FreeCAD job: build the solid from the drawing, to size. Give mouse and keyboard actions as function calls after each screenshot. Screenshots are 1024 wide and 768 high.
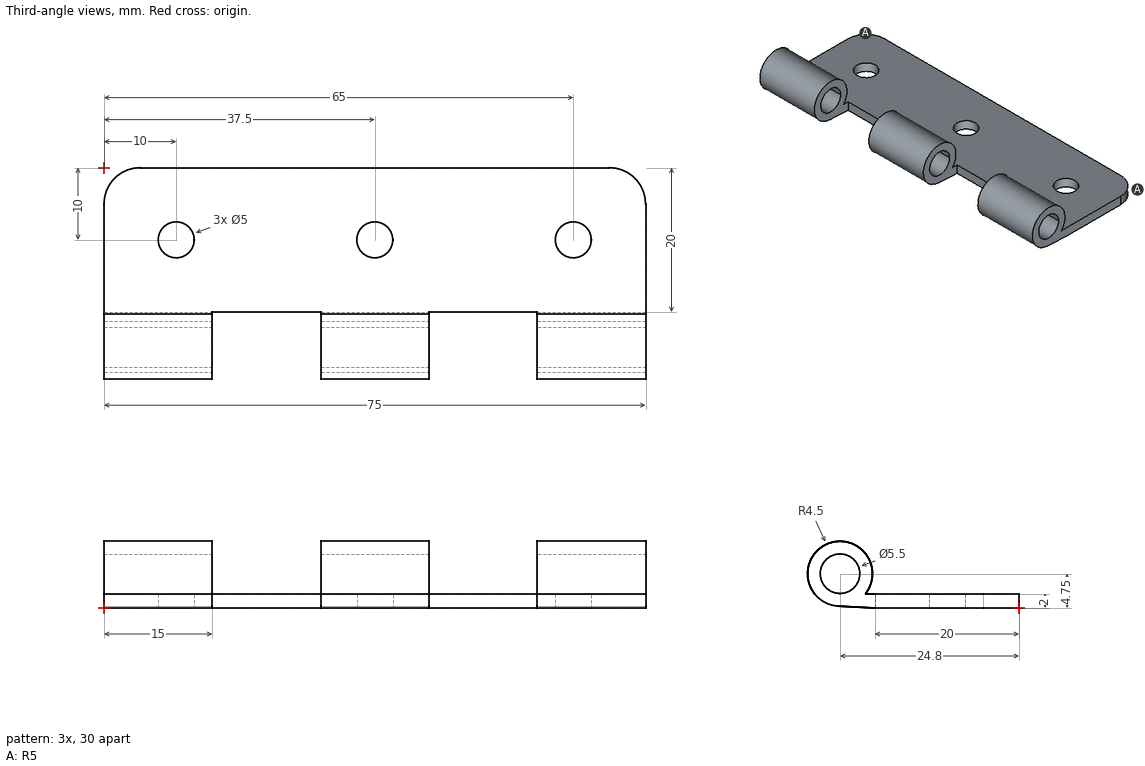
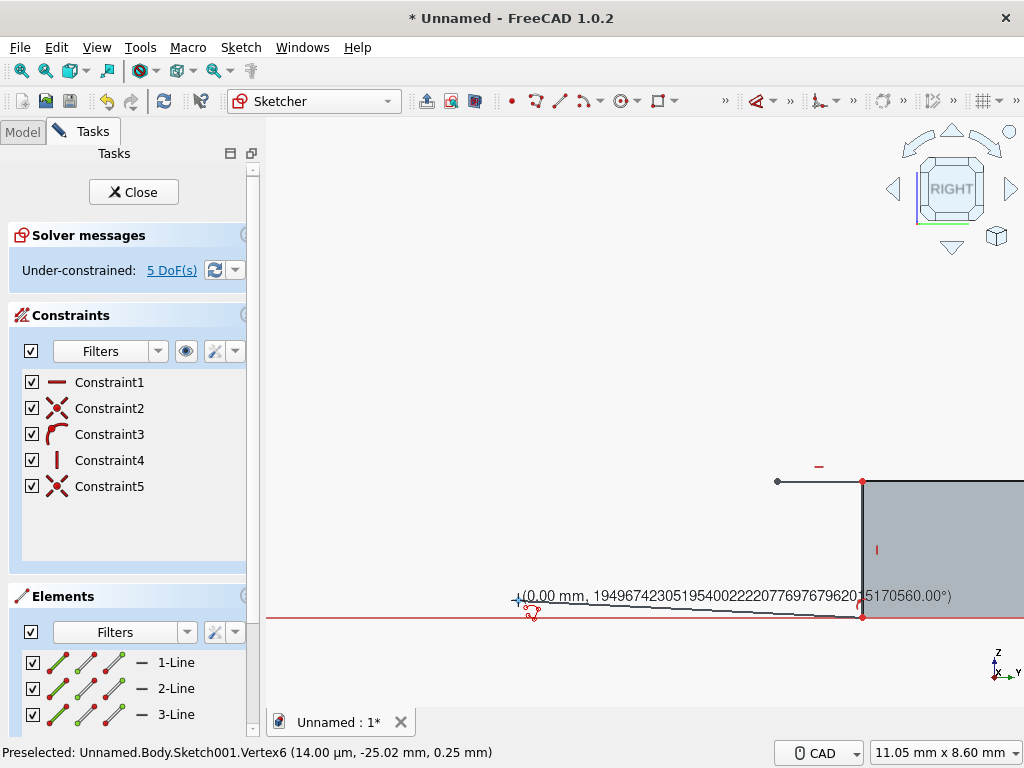
key(g)
key(3)
key(a)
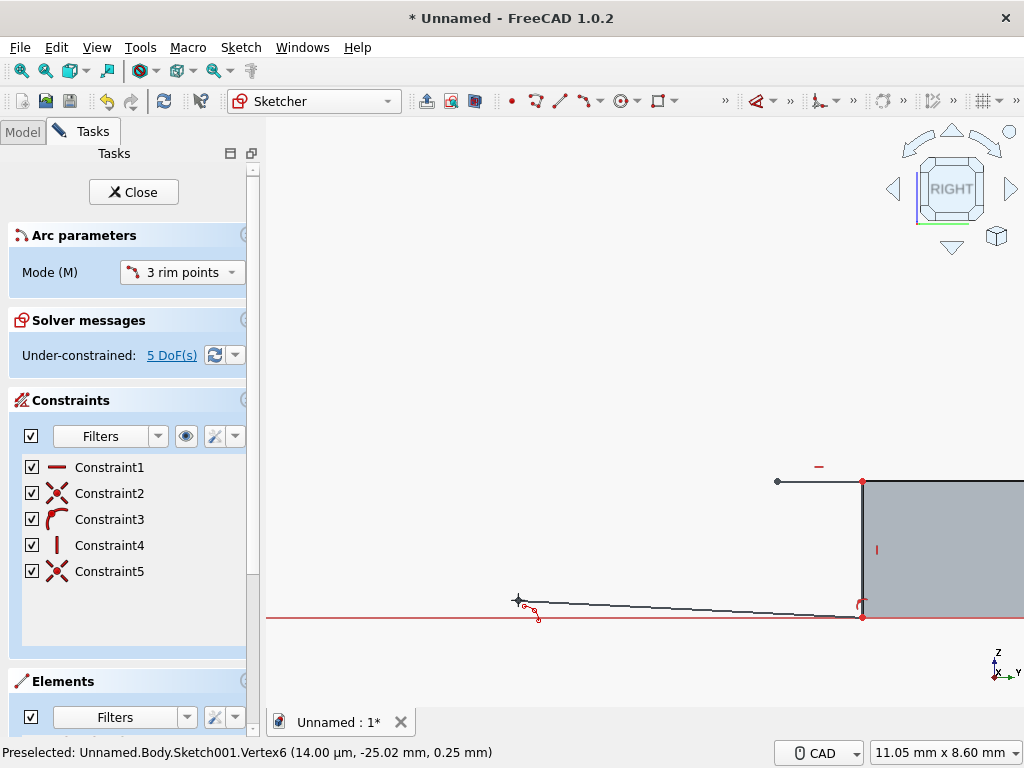
click(518, 601)
click(777, 482)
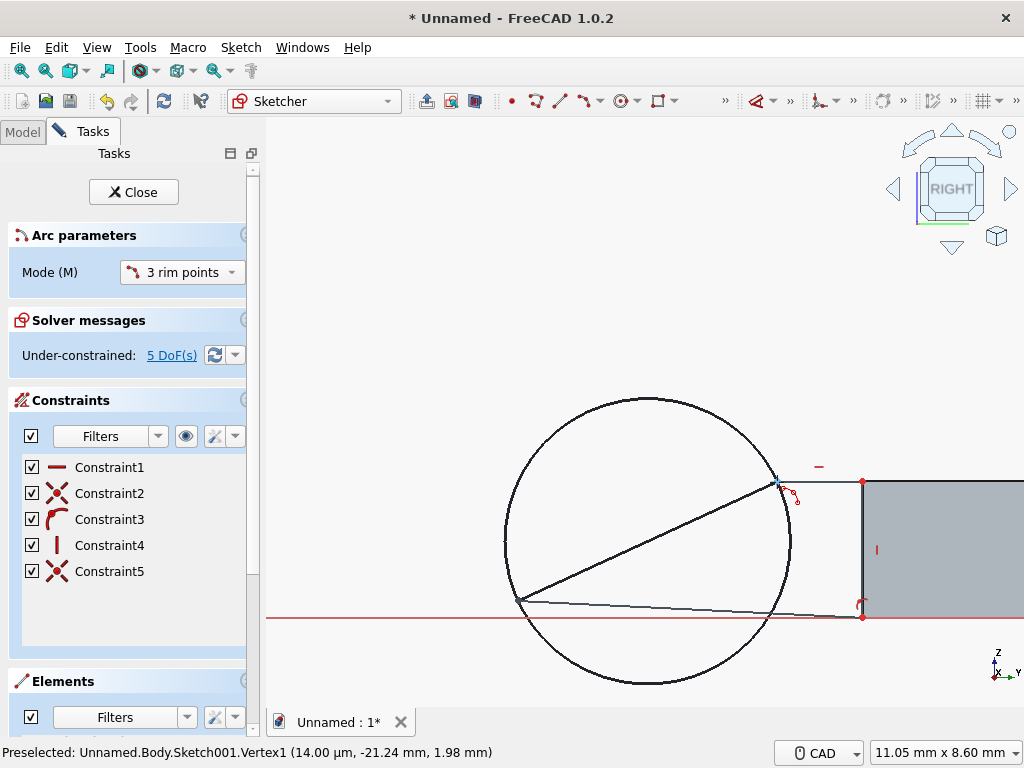
scroll(521, 610, down, 2)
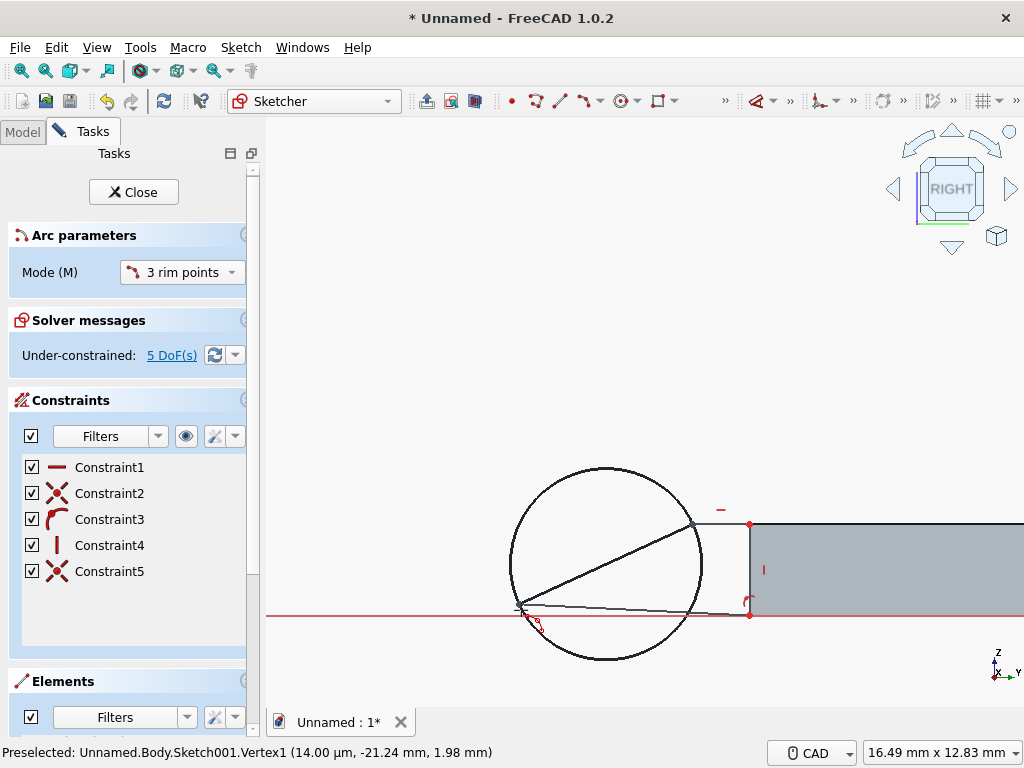
click(443, 209)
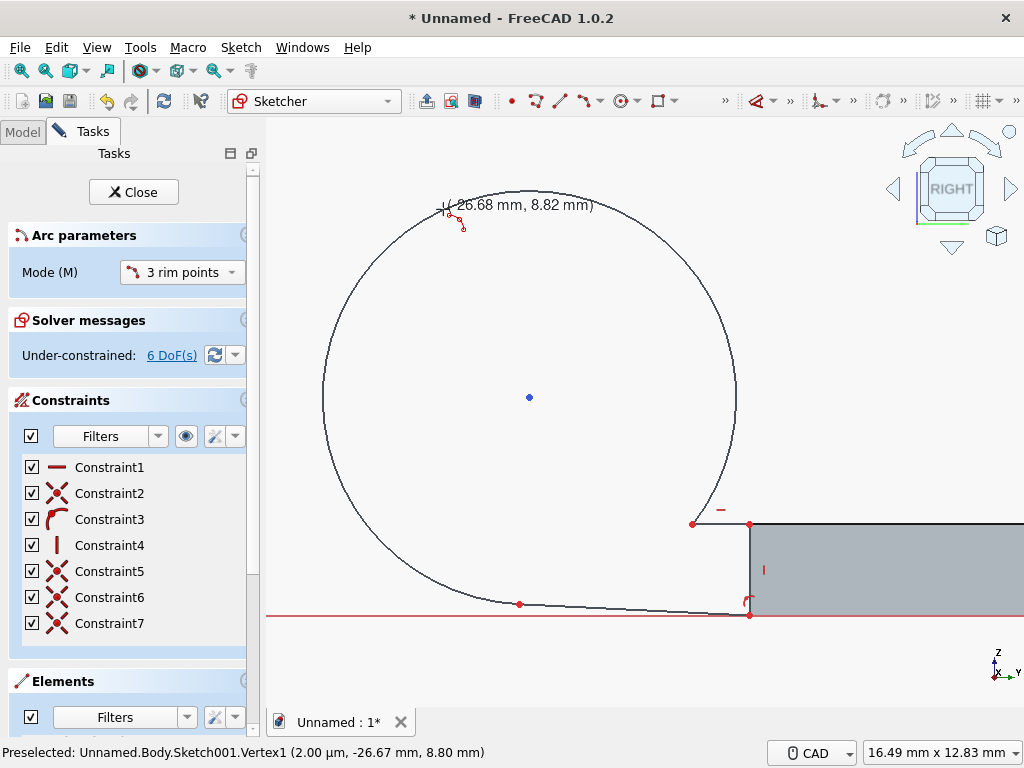
click(622, 102)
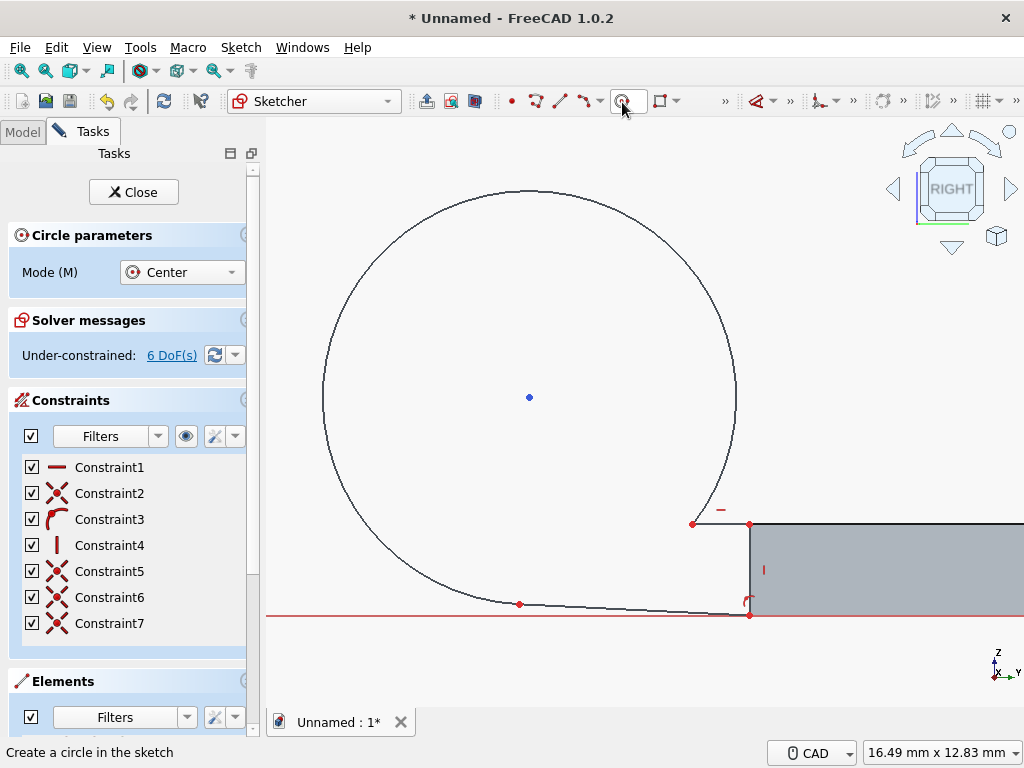
click(529, 397)
move(619, 308)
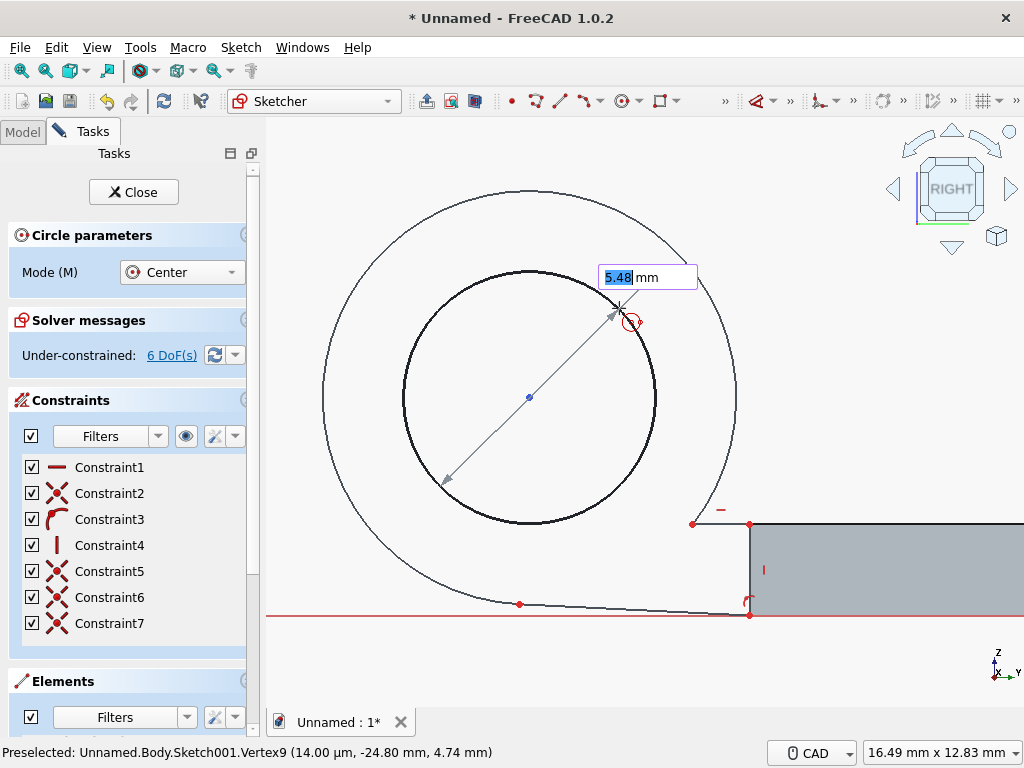
text(5.5)
key(Return)
key(Escape)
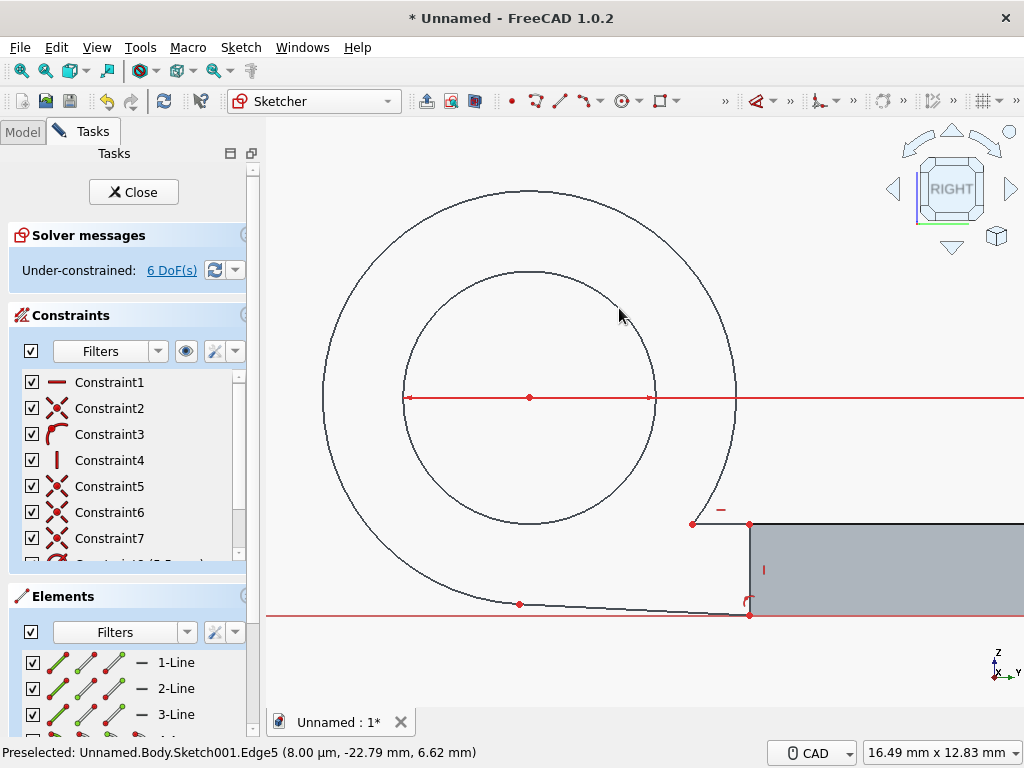
click(681, 612)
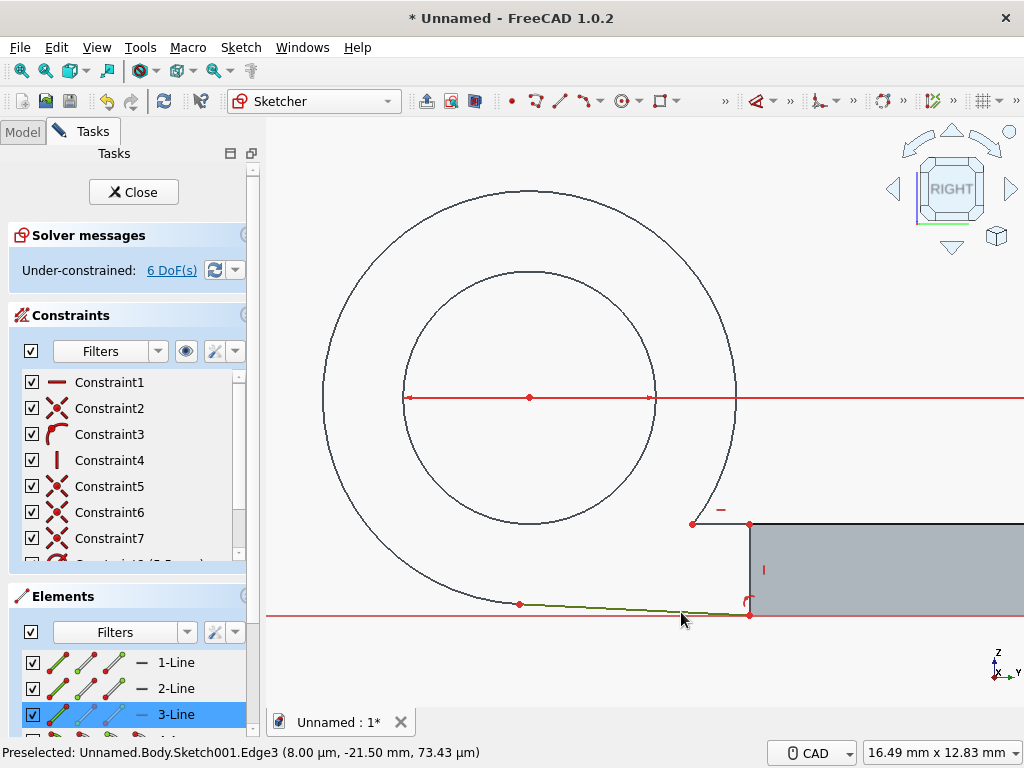
click(652, 231)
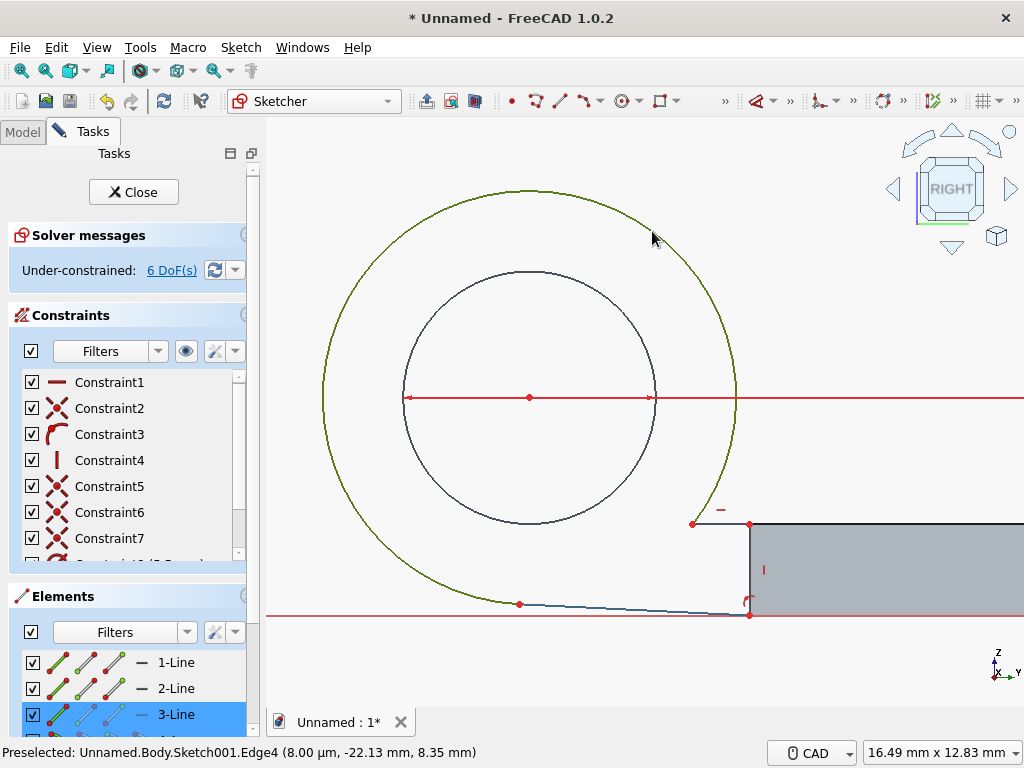
key(t)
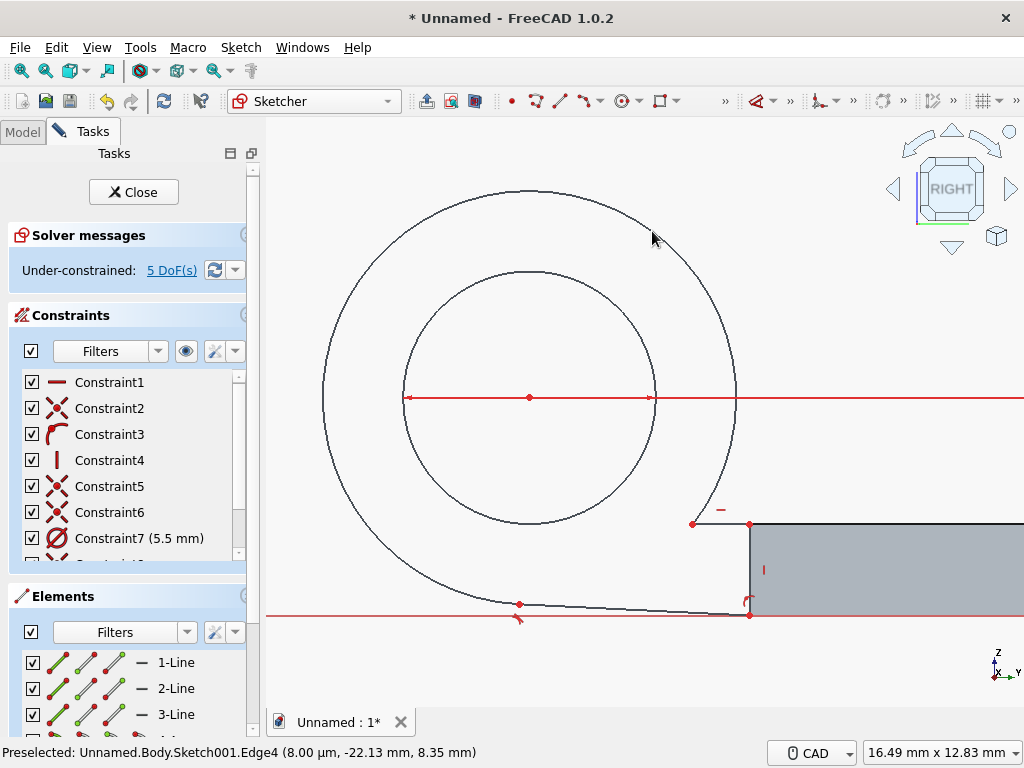
click(756, 102)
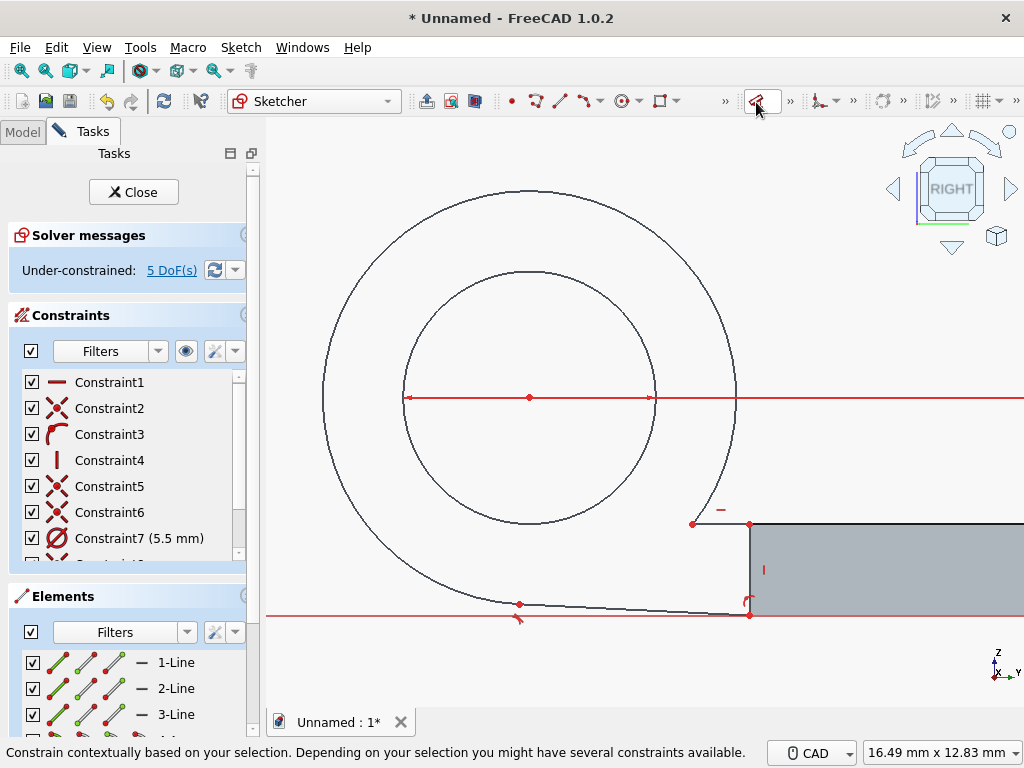
click(652, 231)
click(671, 205)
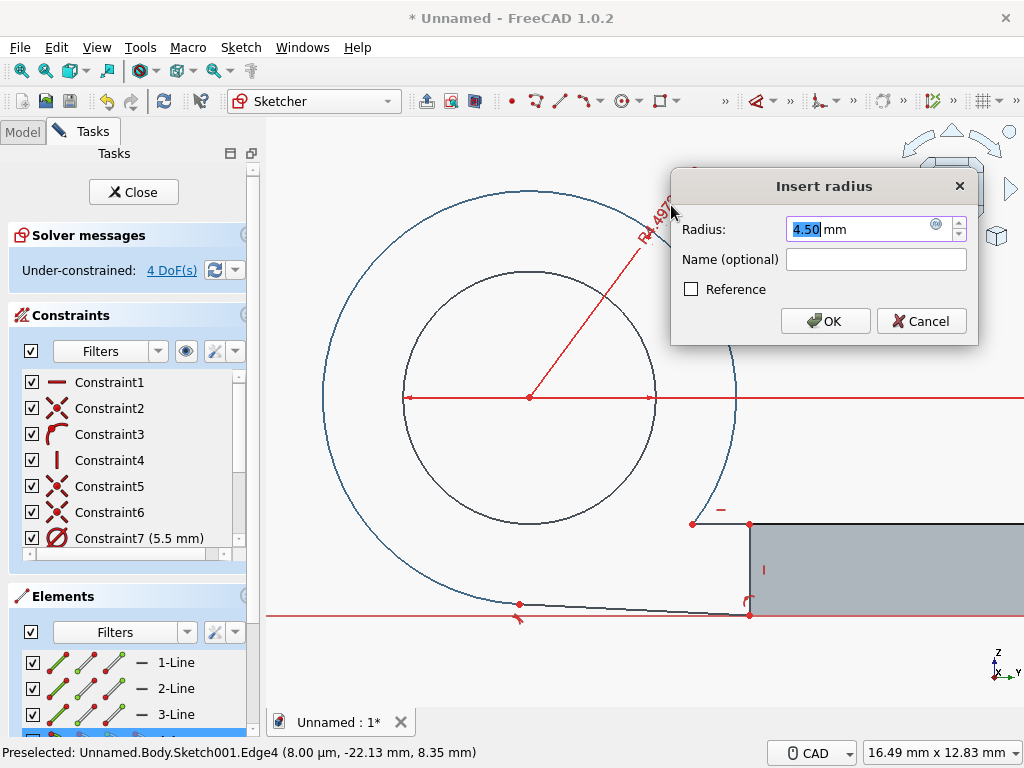
text(4.5)
key(Return)